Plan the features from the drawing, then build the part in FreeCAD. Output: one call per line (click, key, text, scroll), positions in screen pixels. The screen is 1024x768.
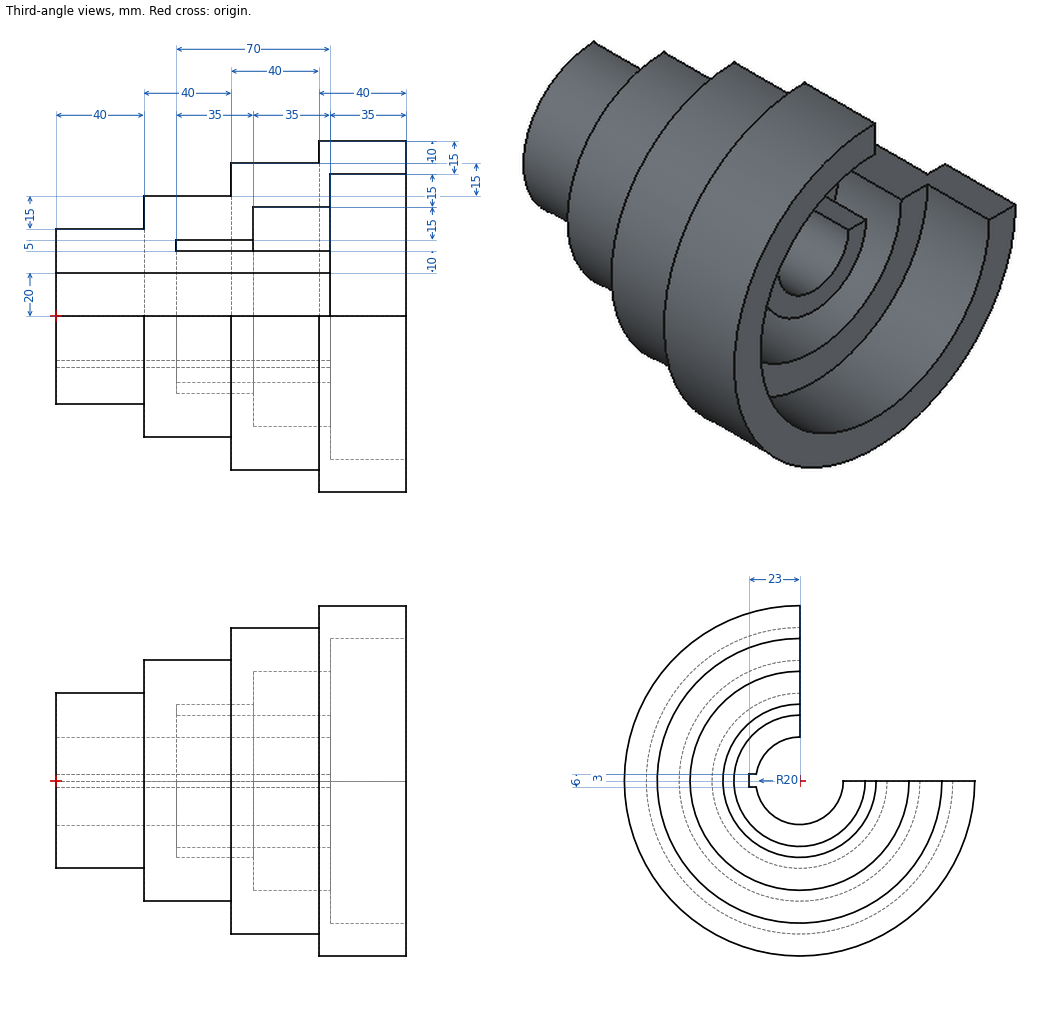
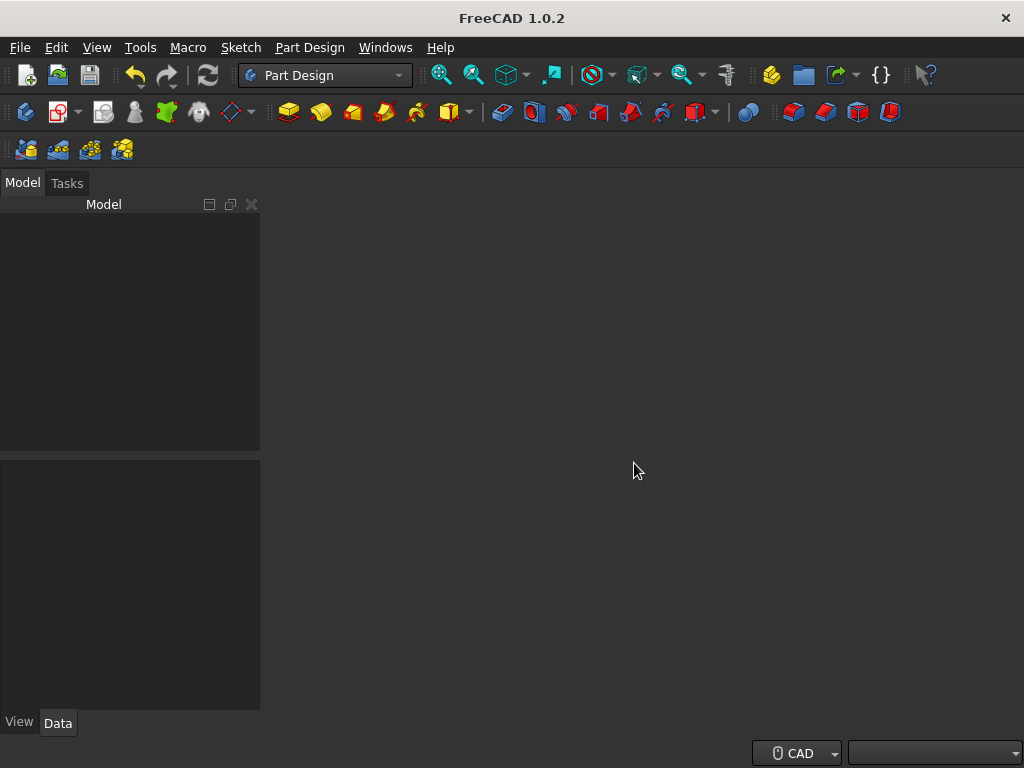
key(ctrl+n)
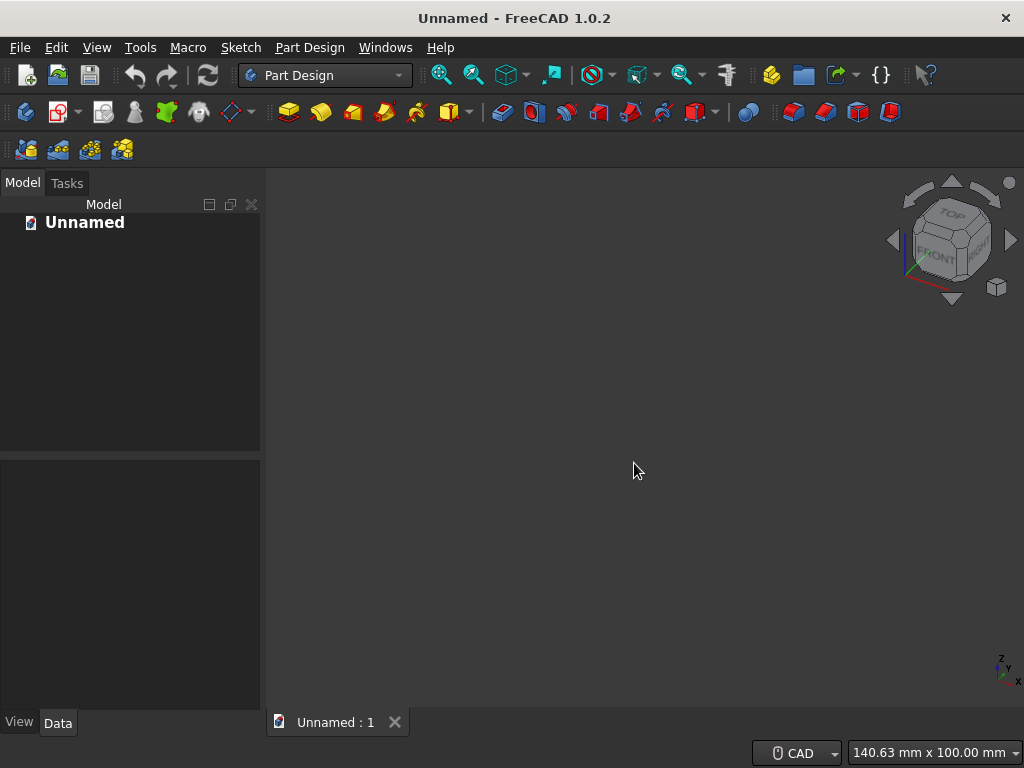
click(58, 112)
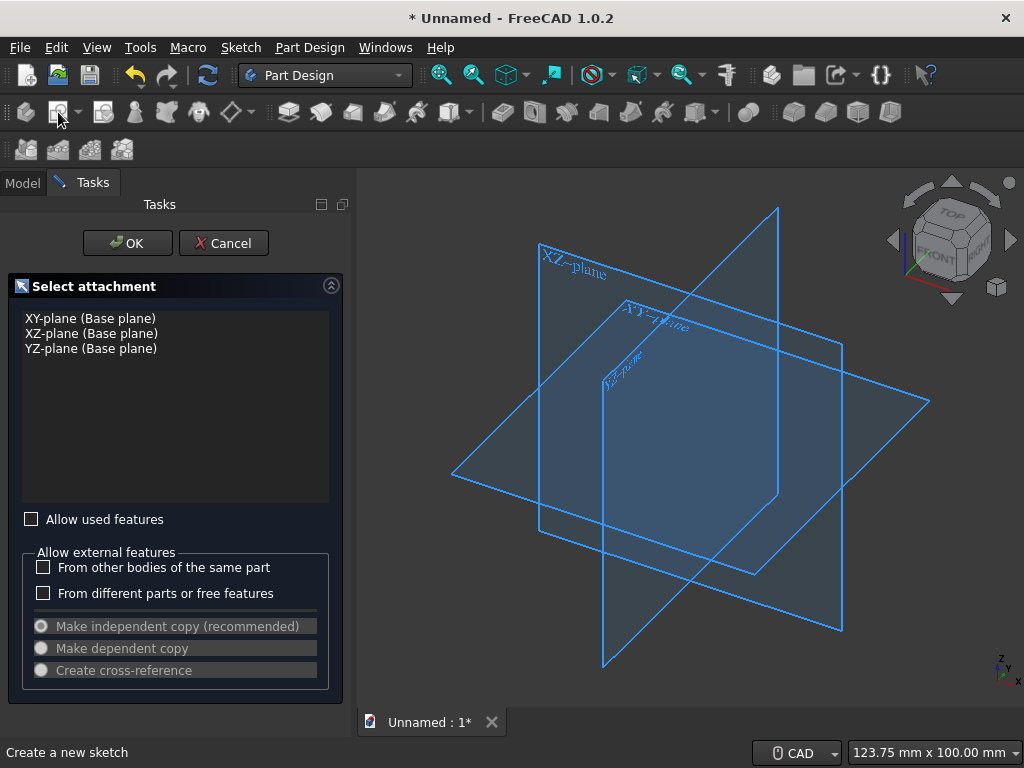
click(82, 318)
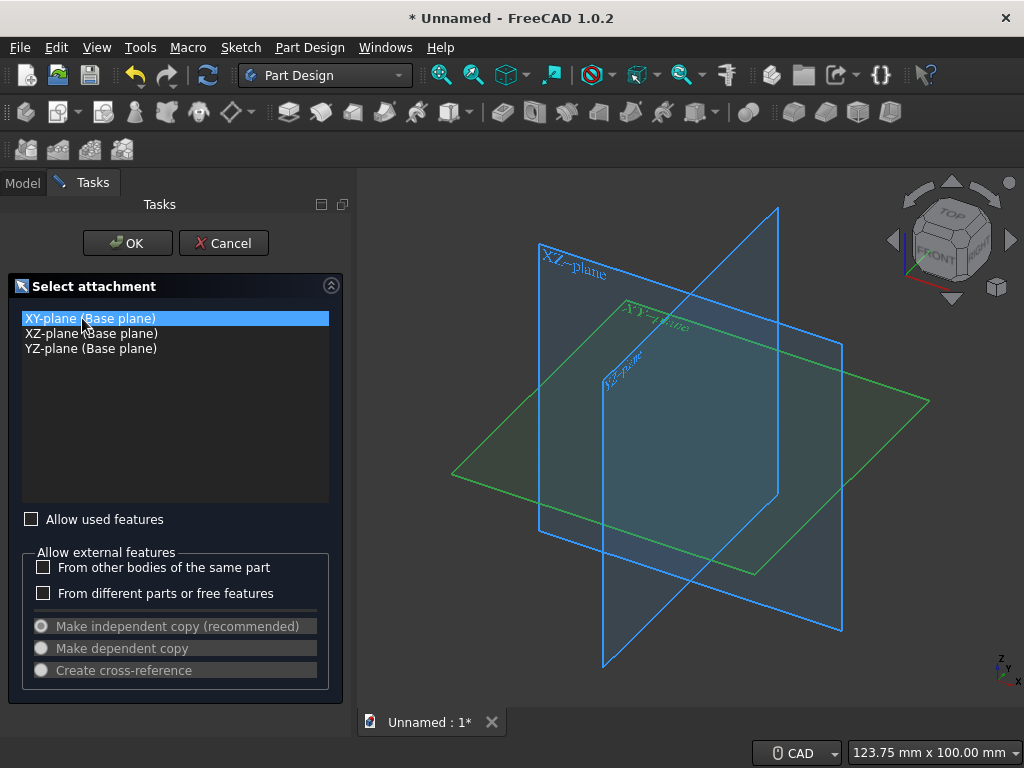
click(128, 243)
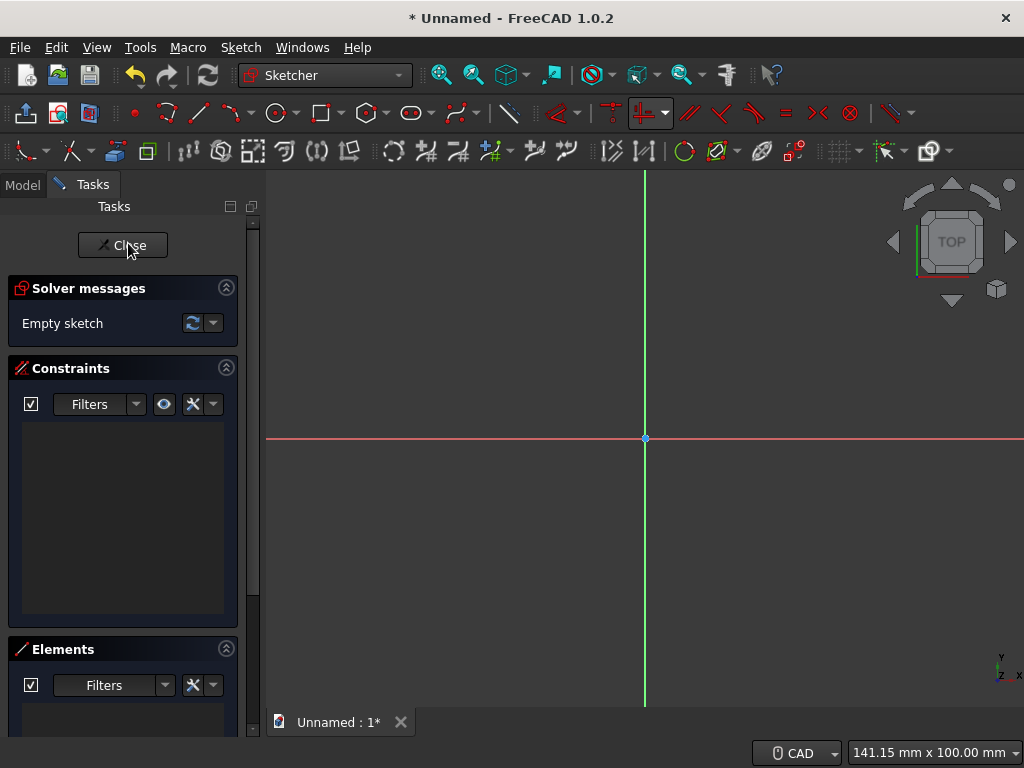
scroll(294, 564, down, 5)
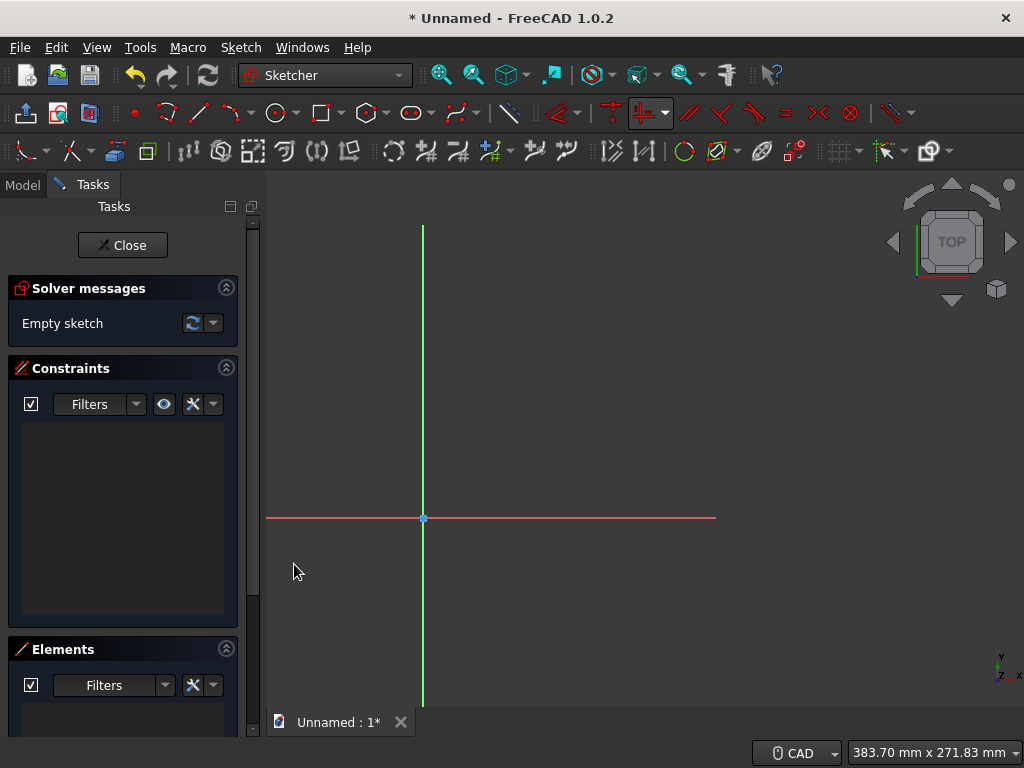
click(168, 114)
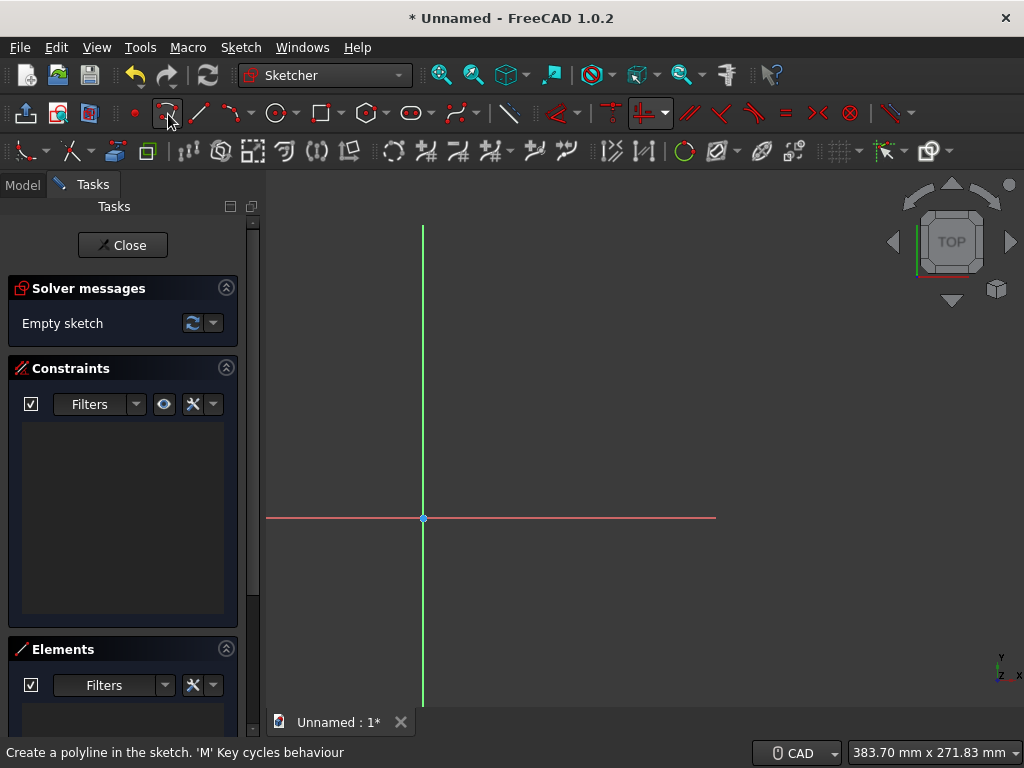
click(423, 479)
click(670, 479)
click(670, 459)
click(532, 459)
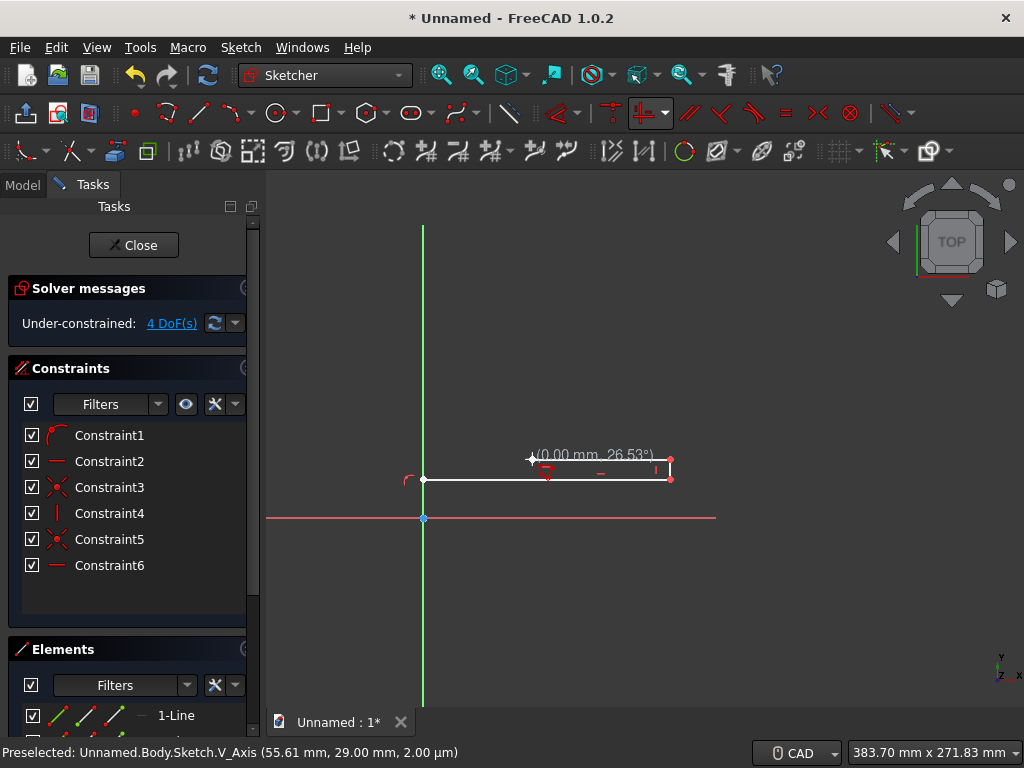
scroll(532, 449, up, 3)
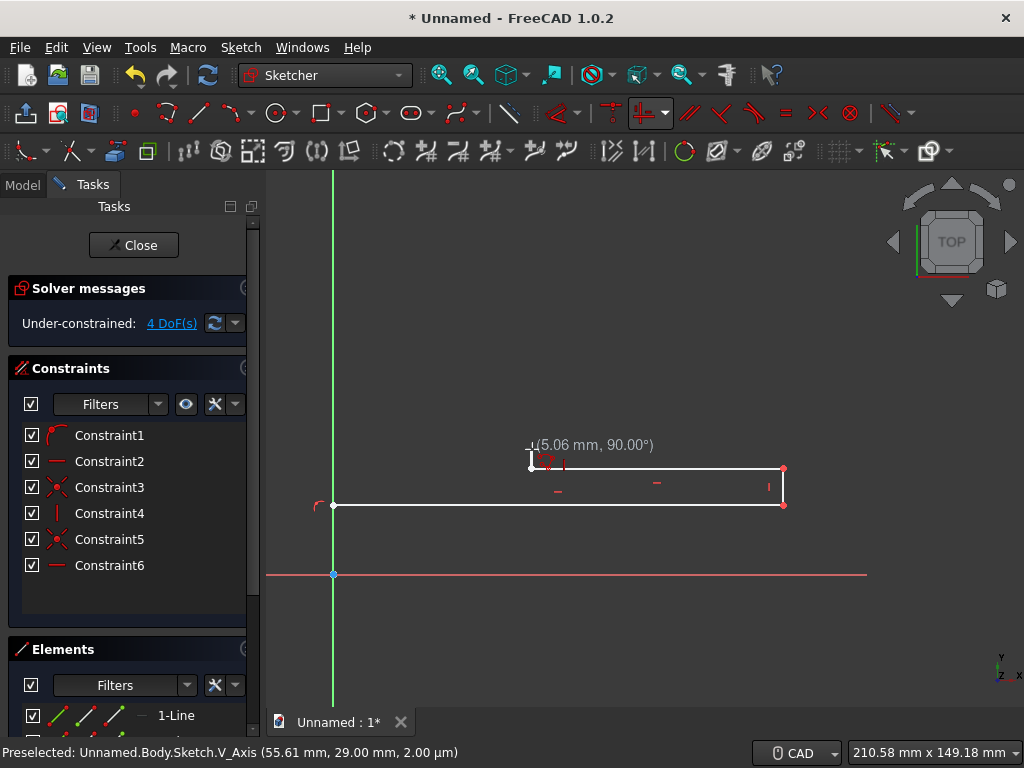
click(532, 449)
click(657, 449)
click(657, 395)
click(783, 395)
click(783, 341)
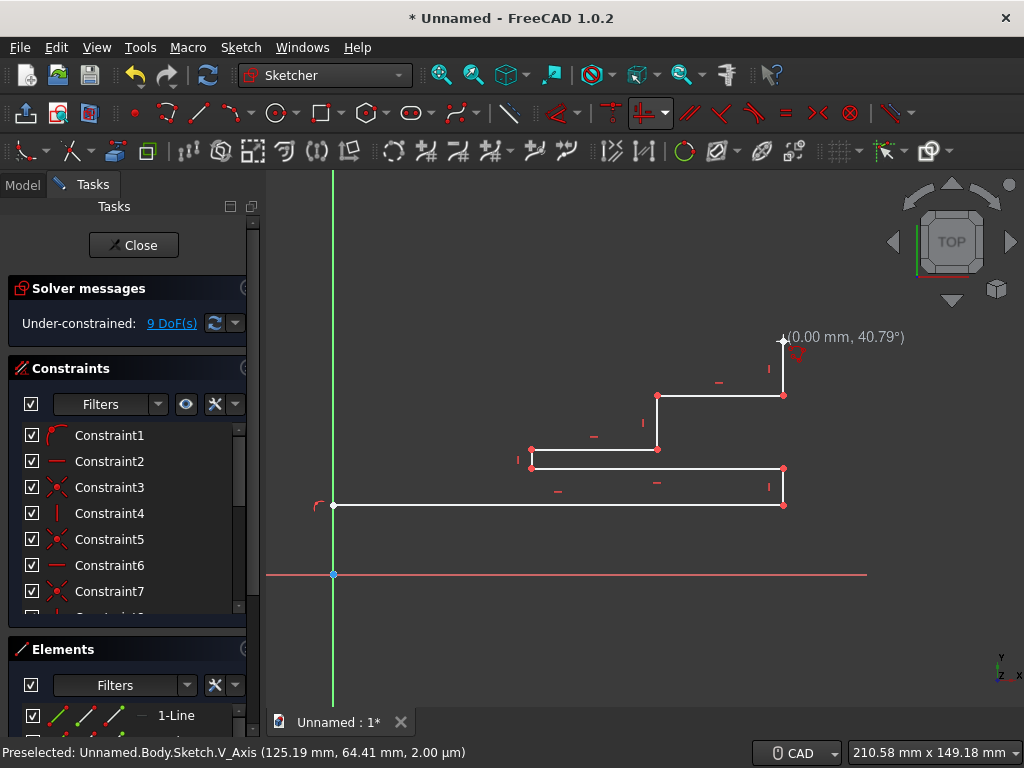
scroll(485, 454, down, 2)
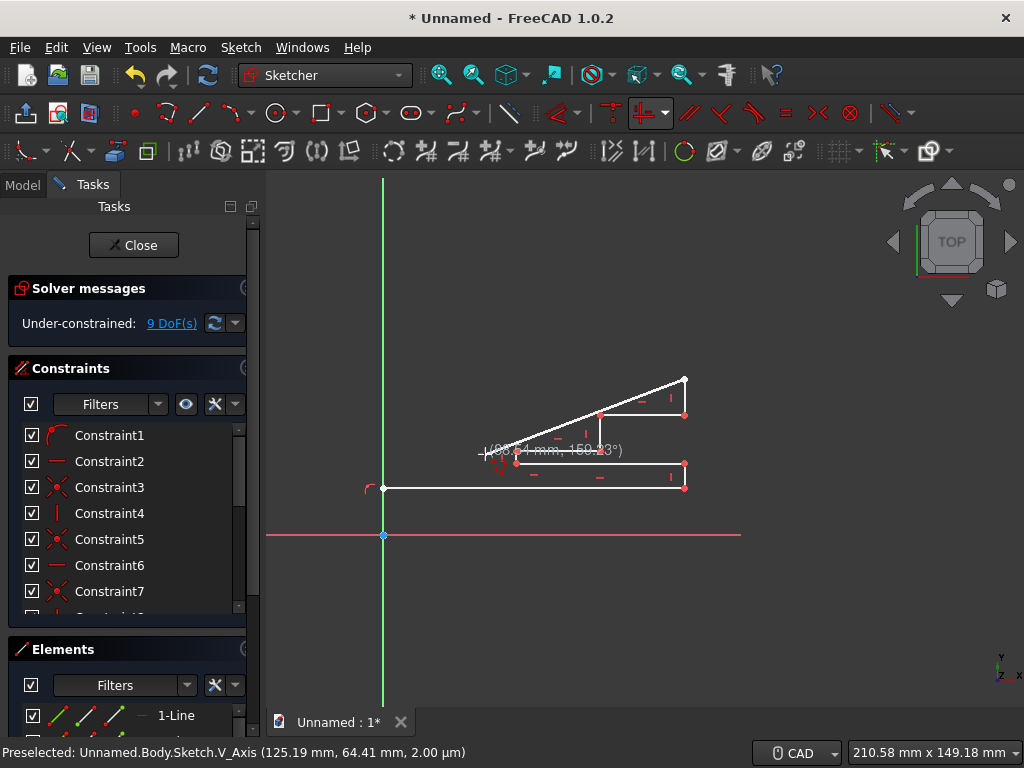
click(770, 378)
click(770, 342)
click(673, 342)
click(673, 366)
click(576, 366)
click(576, 402)
click(480, 402)
click(480, 439)
click(392, 439)
click(383, 488)
key(Escape)
key(Escape)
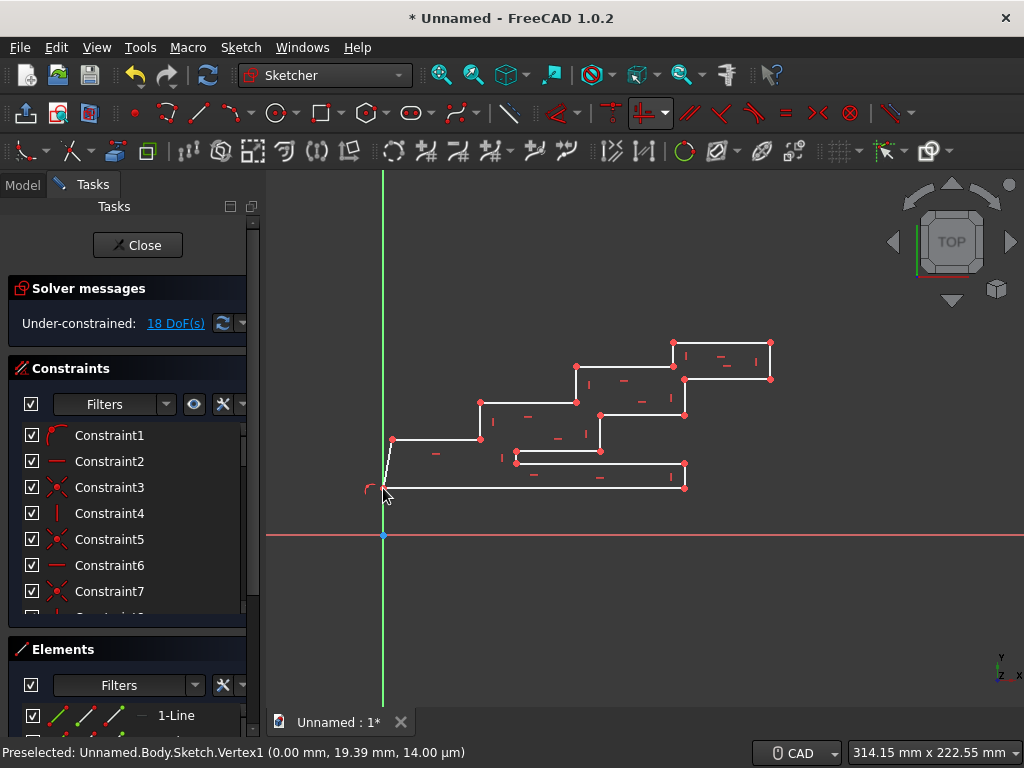
click(386, 474)